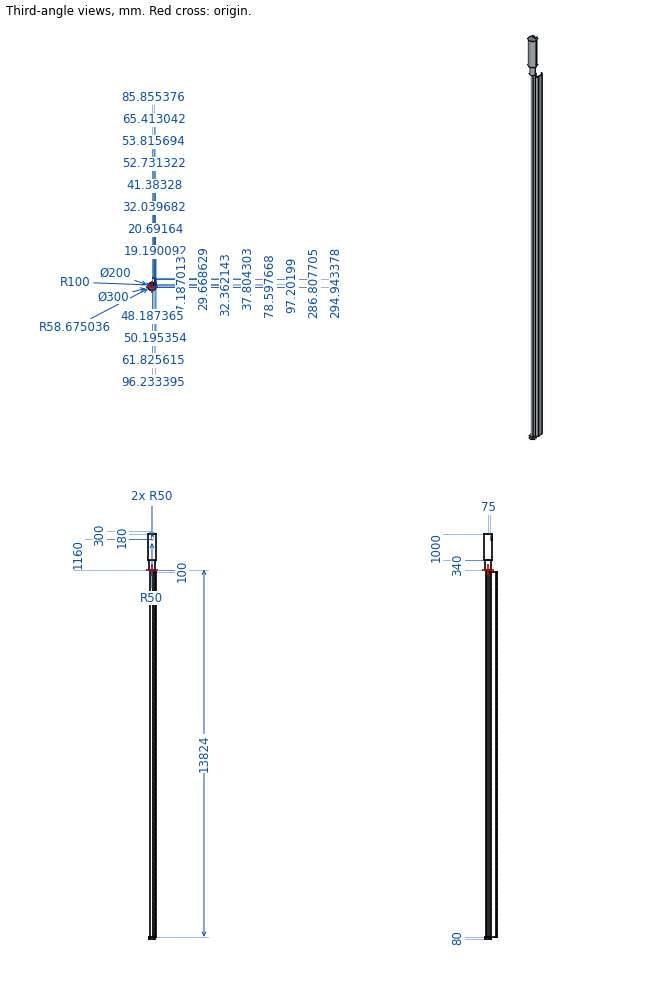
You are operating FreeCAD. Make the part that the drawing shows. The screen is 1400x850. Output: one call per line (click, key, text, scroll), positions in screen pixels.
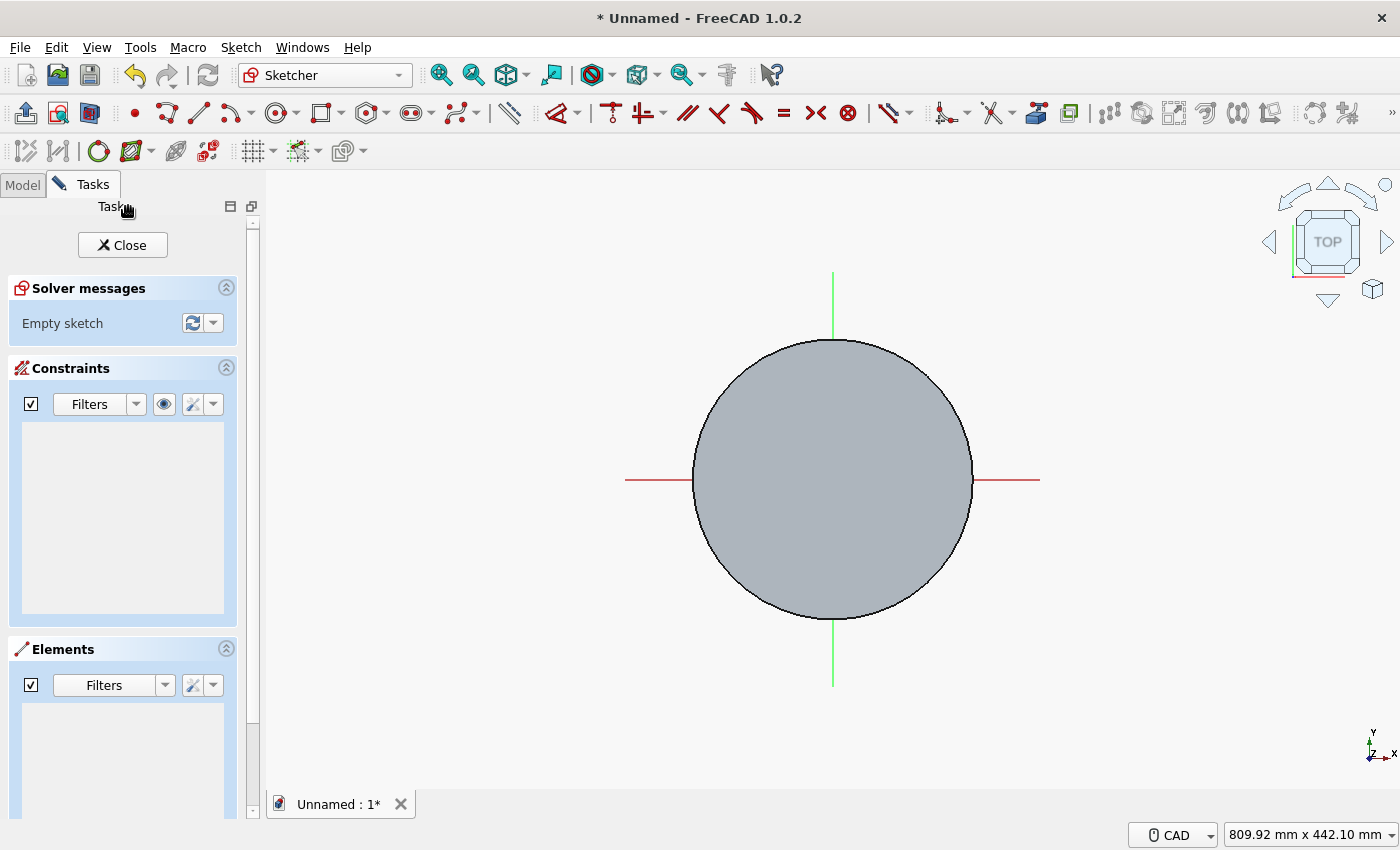
key(q)
key(s)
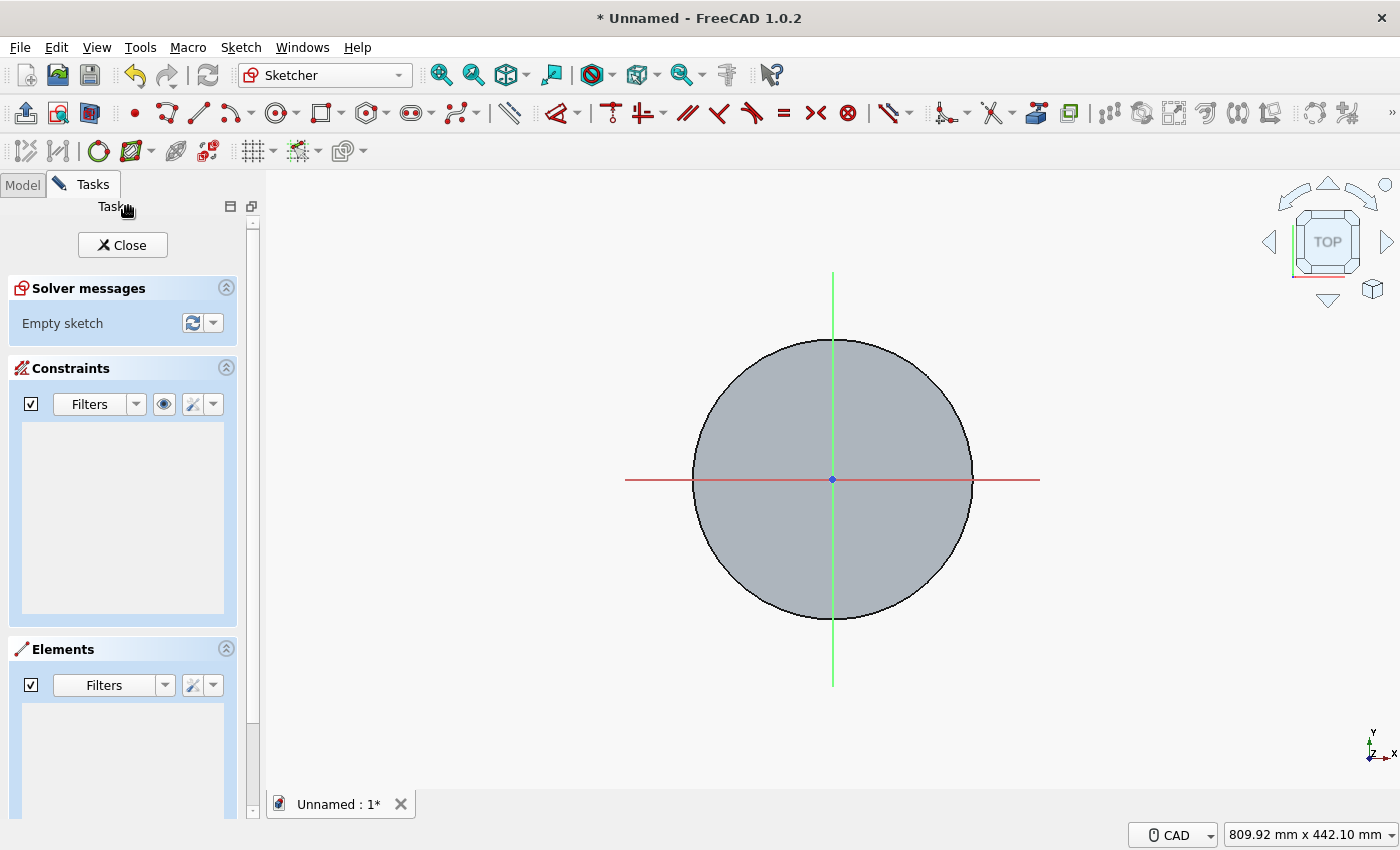
scroll(491, 761, down, 2)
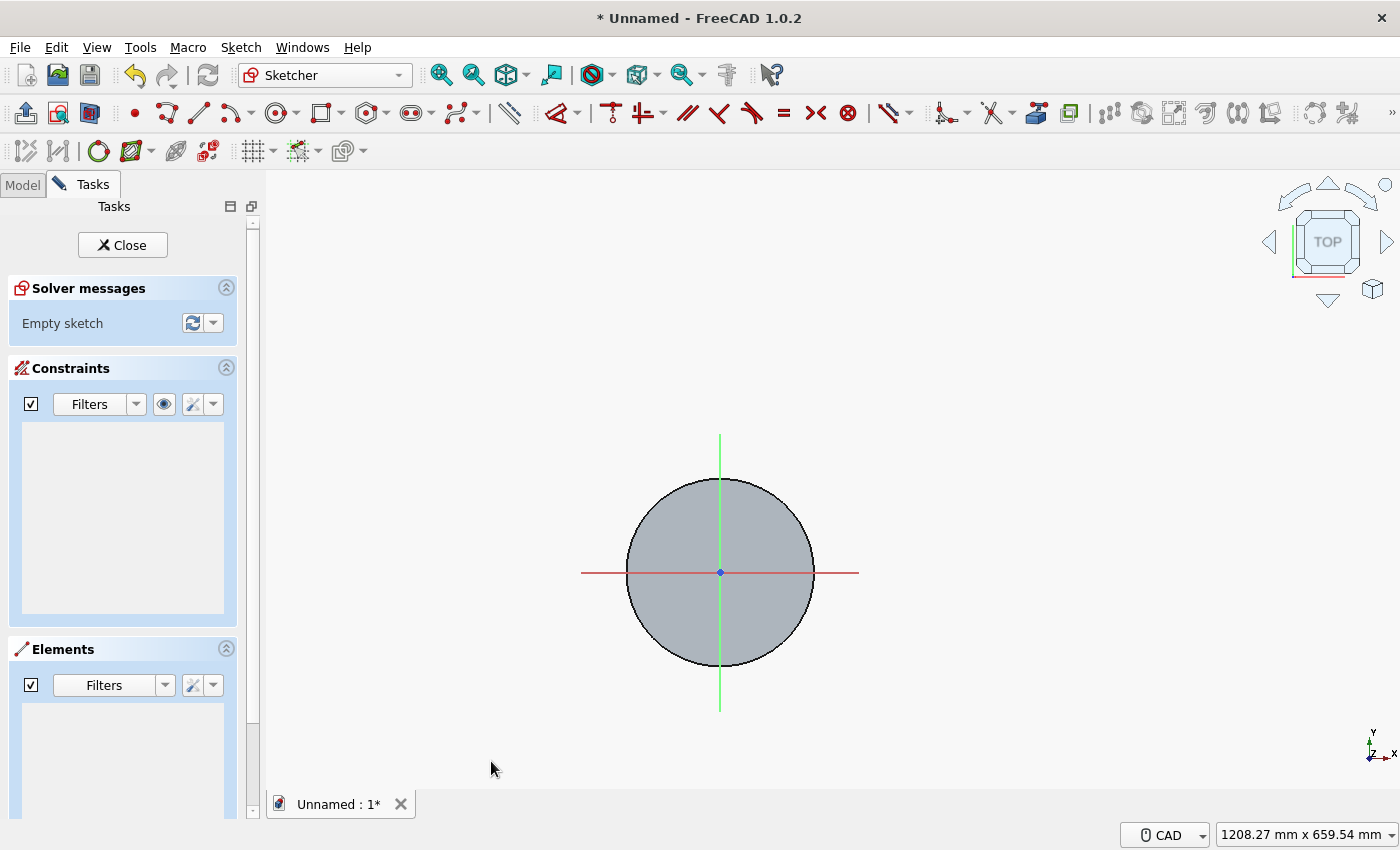
click(168, 114)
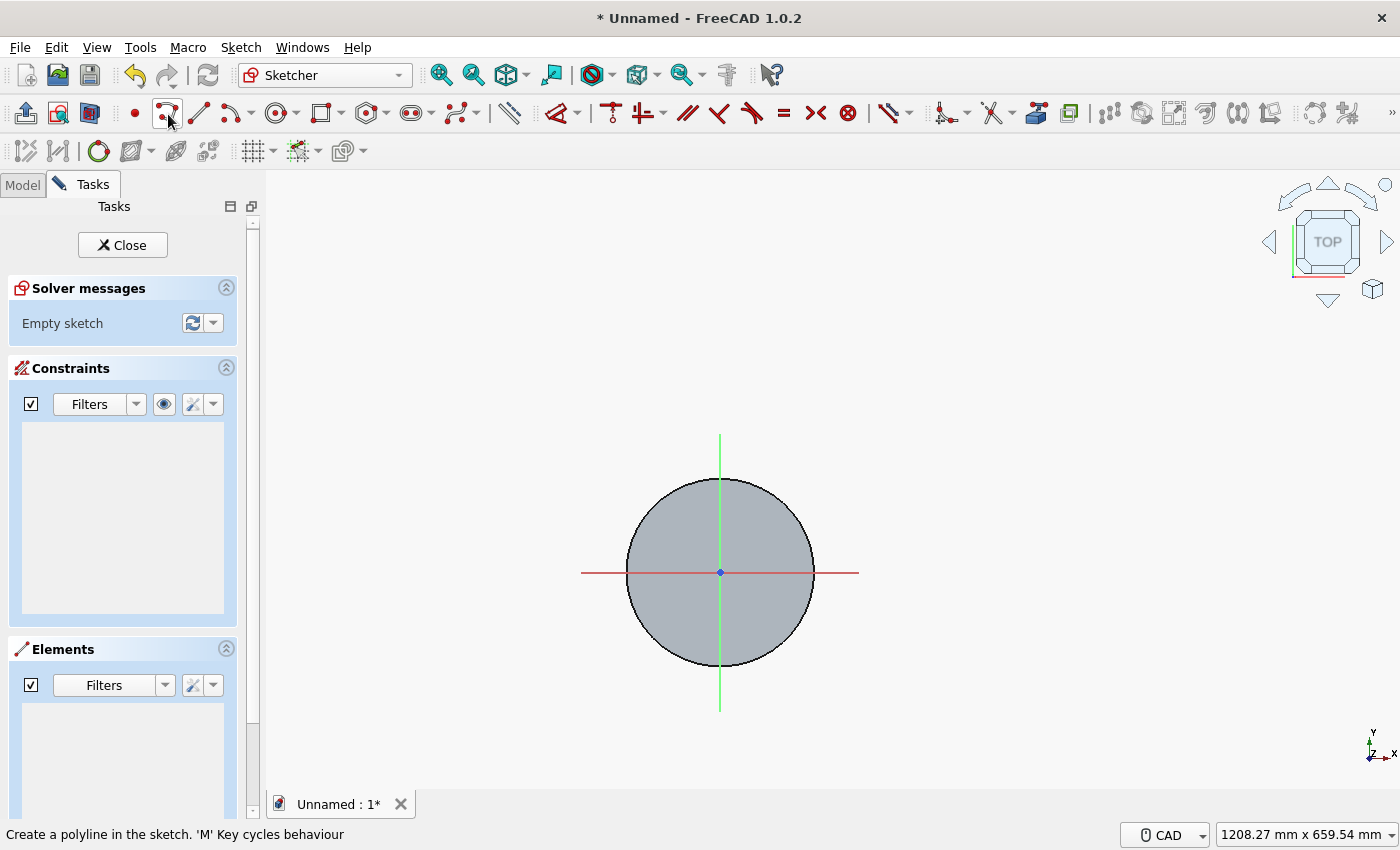
click(720, 518)
click(778, 499)
click(840, 468)
click(820, 303)
click(771, 268)
click(801, 268)
click(840, 296)
click(858, 481)
click(811, 547)
click(765, 604)
right_click(765, 604)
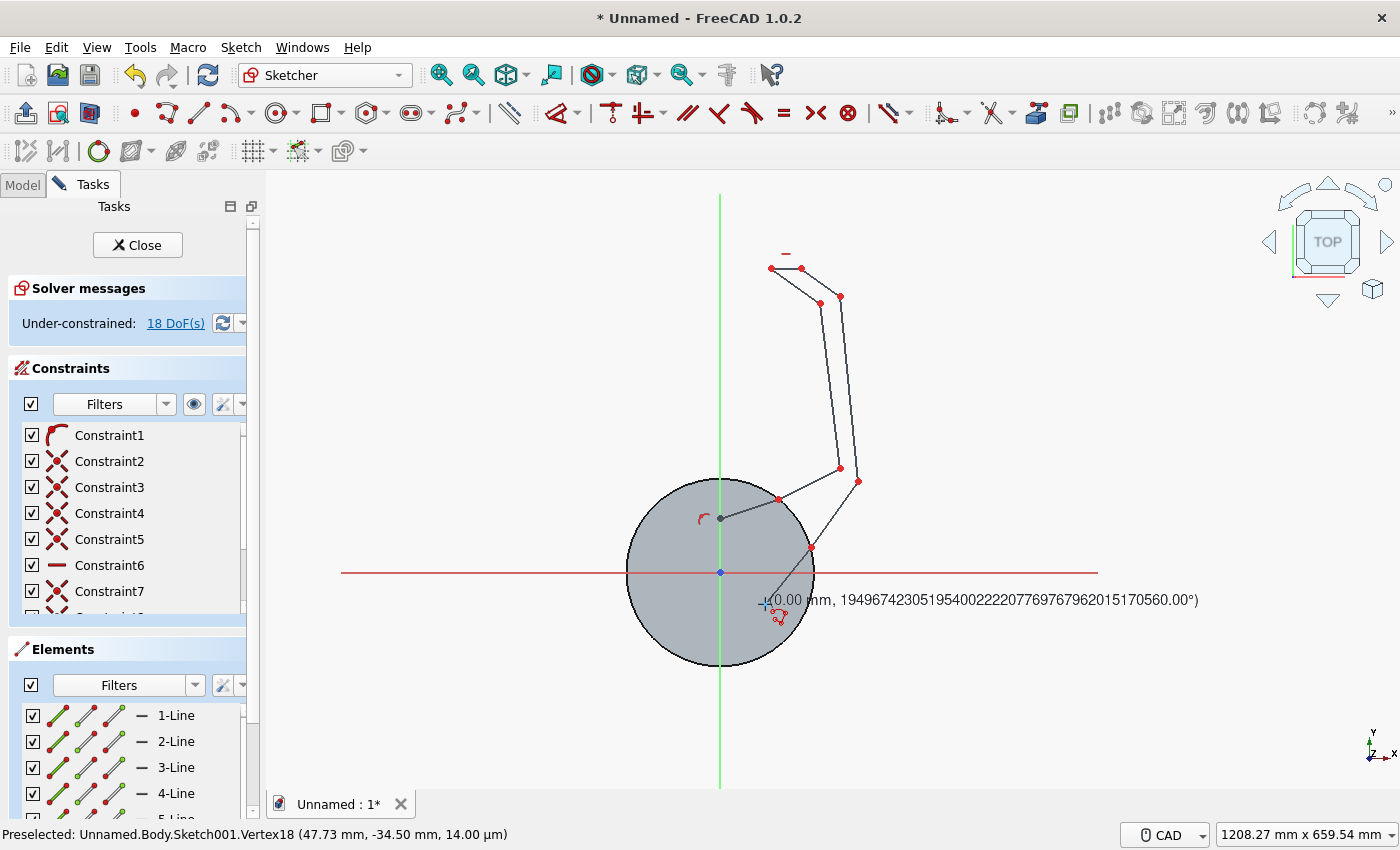
key(g)
key(3)
key(a)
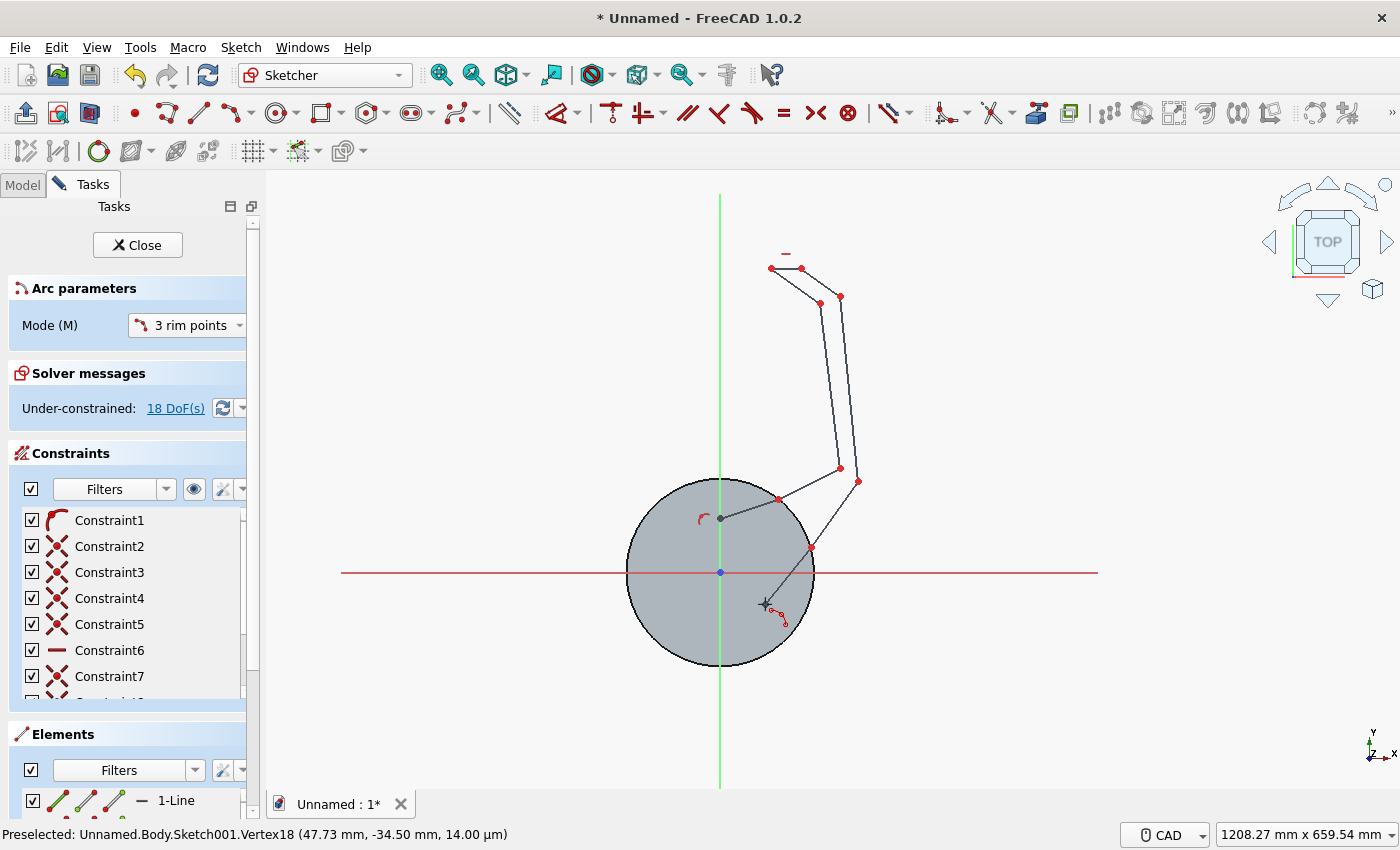
click(765, 605)
click(720, 519)
click(671, 598)
key(Escape)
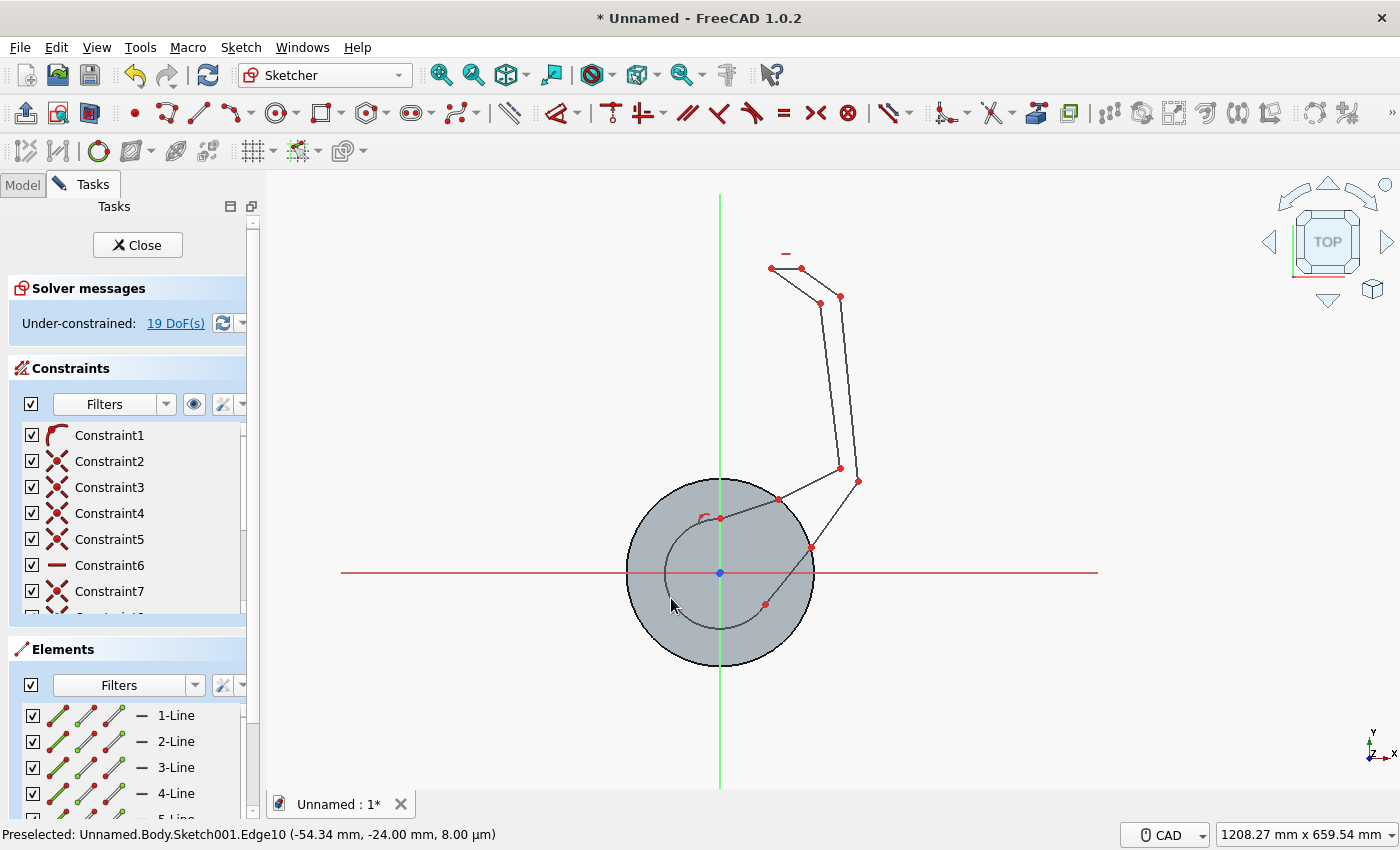
drag(710, 563, 730, 584)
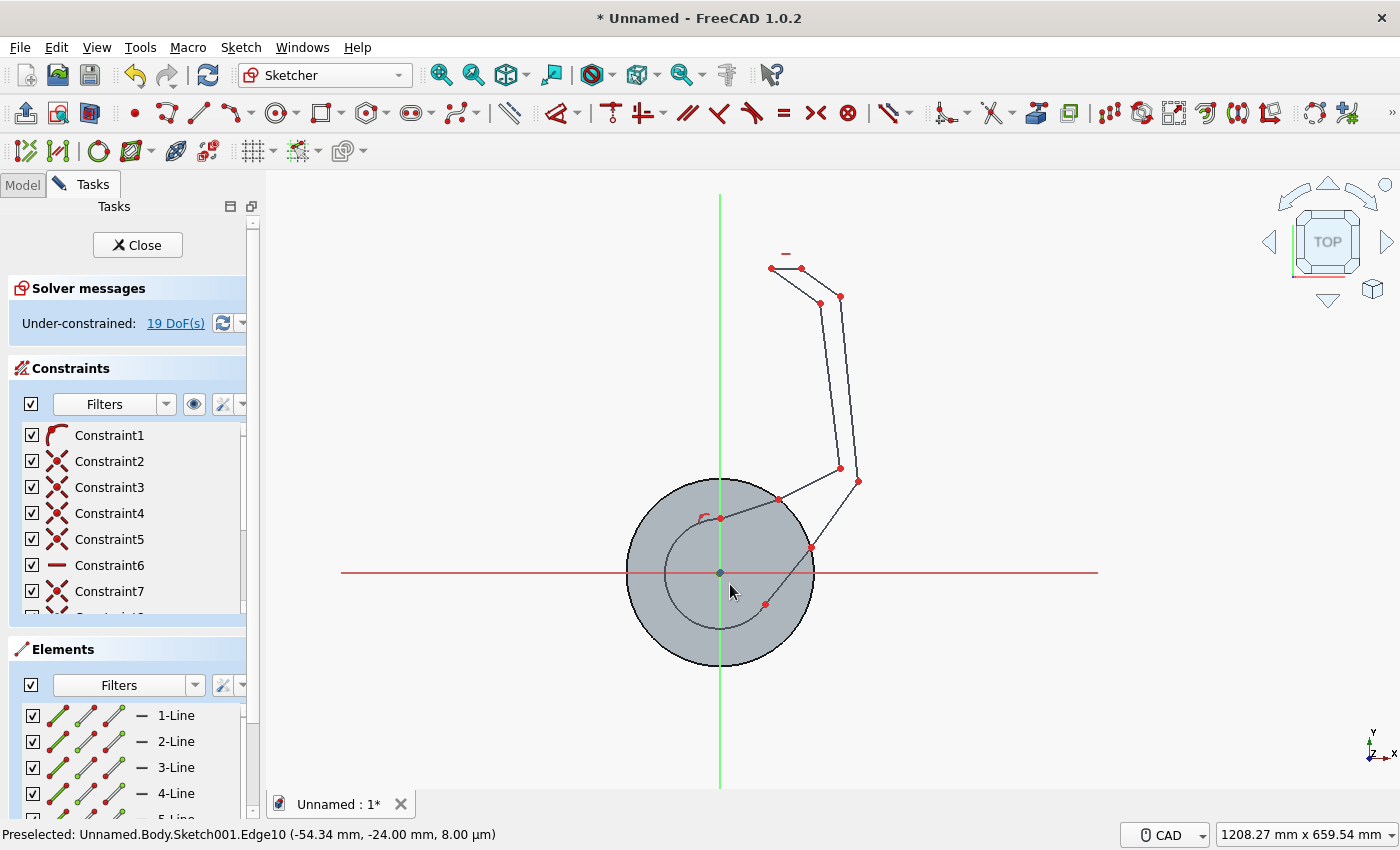
click(612, 114)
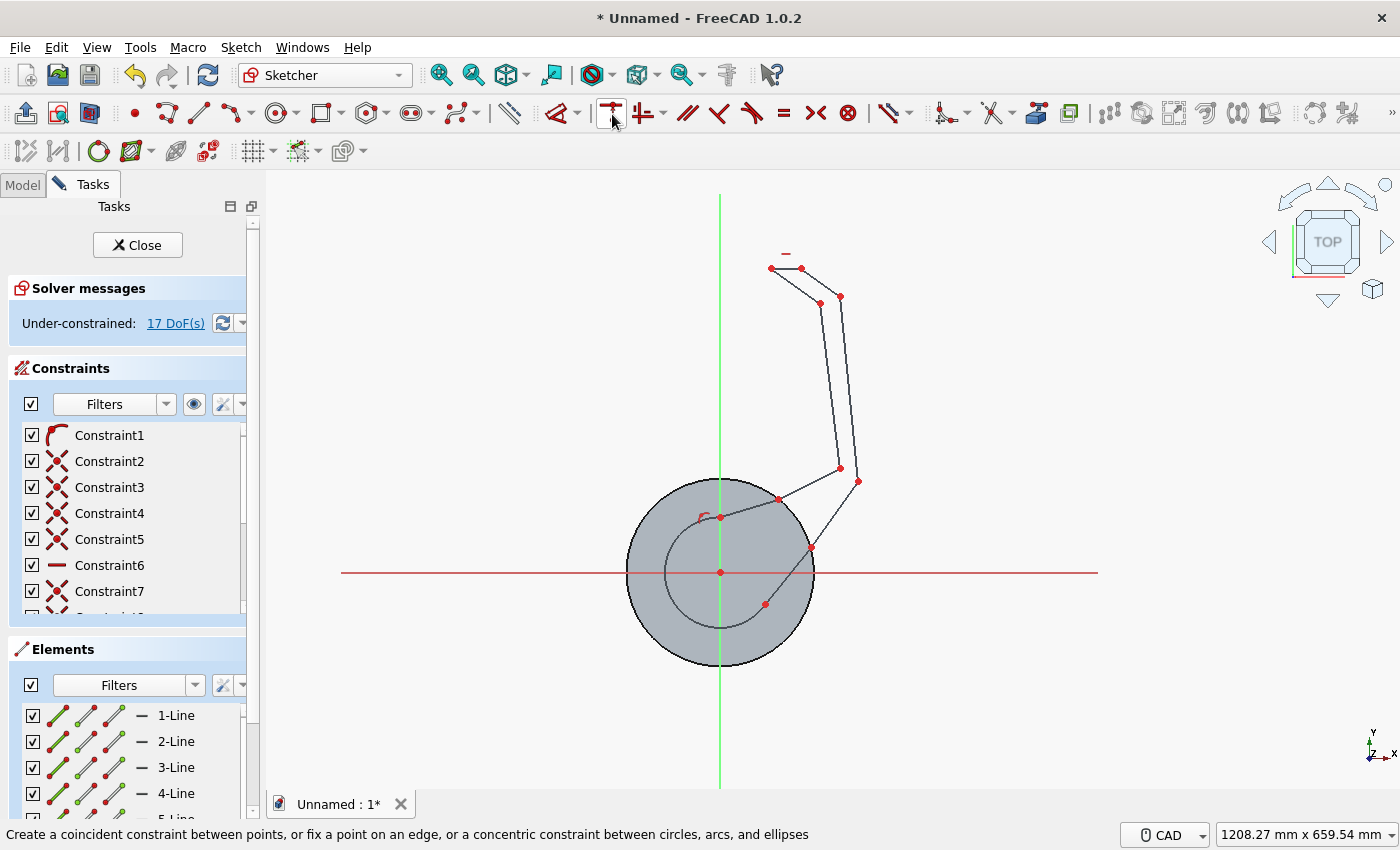
click(556, 114)